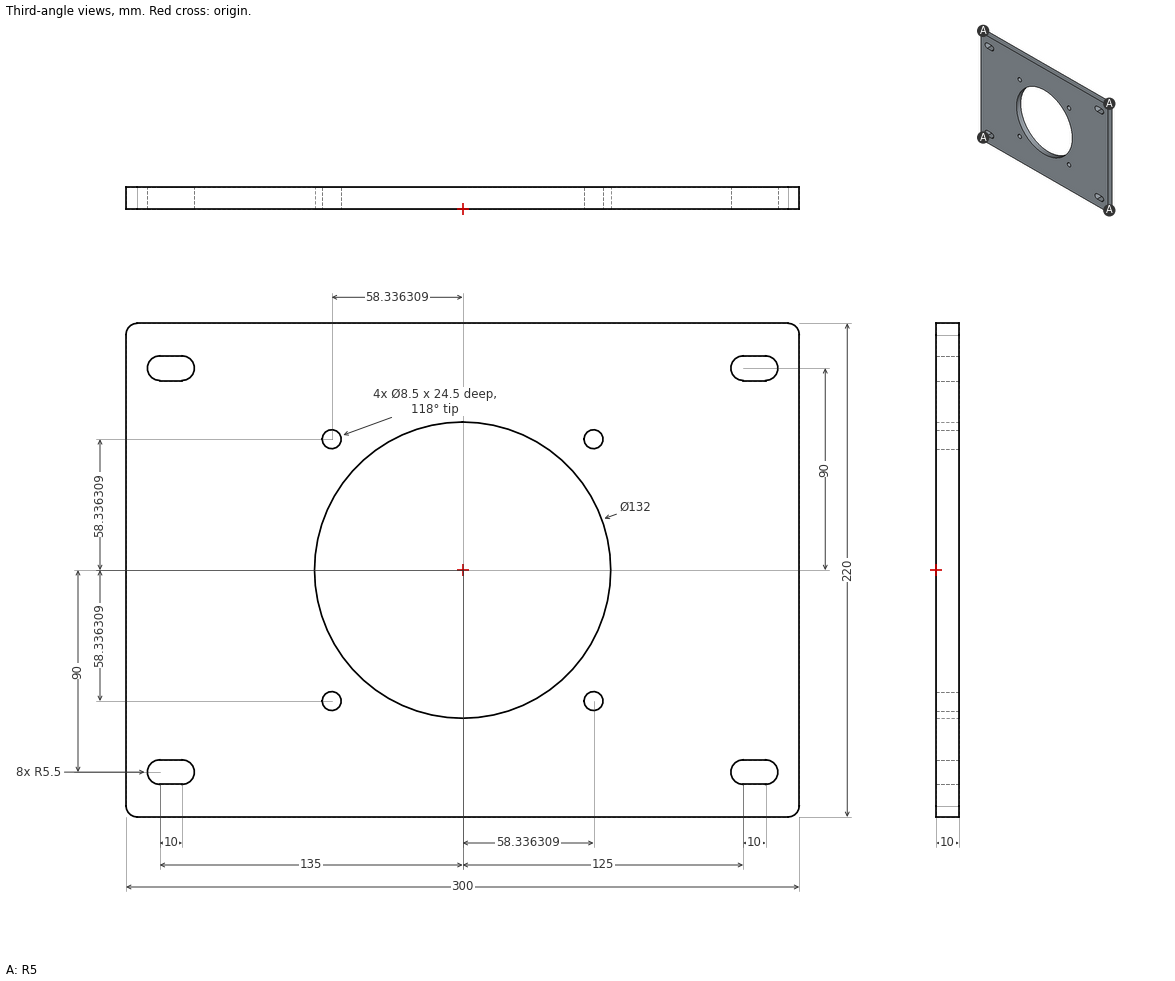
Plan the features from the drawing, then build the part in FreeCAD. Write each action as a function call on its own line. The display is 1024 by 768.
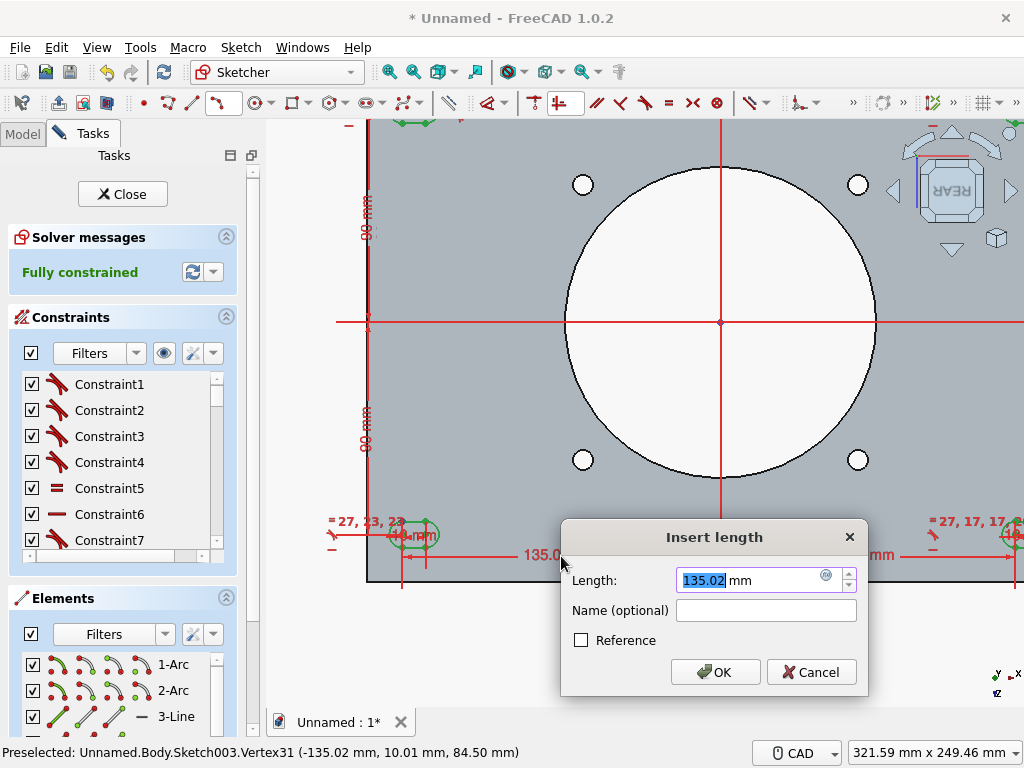
text(135)
key(Return)
key(Escape)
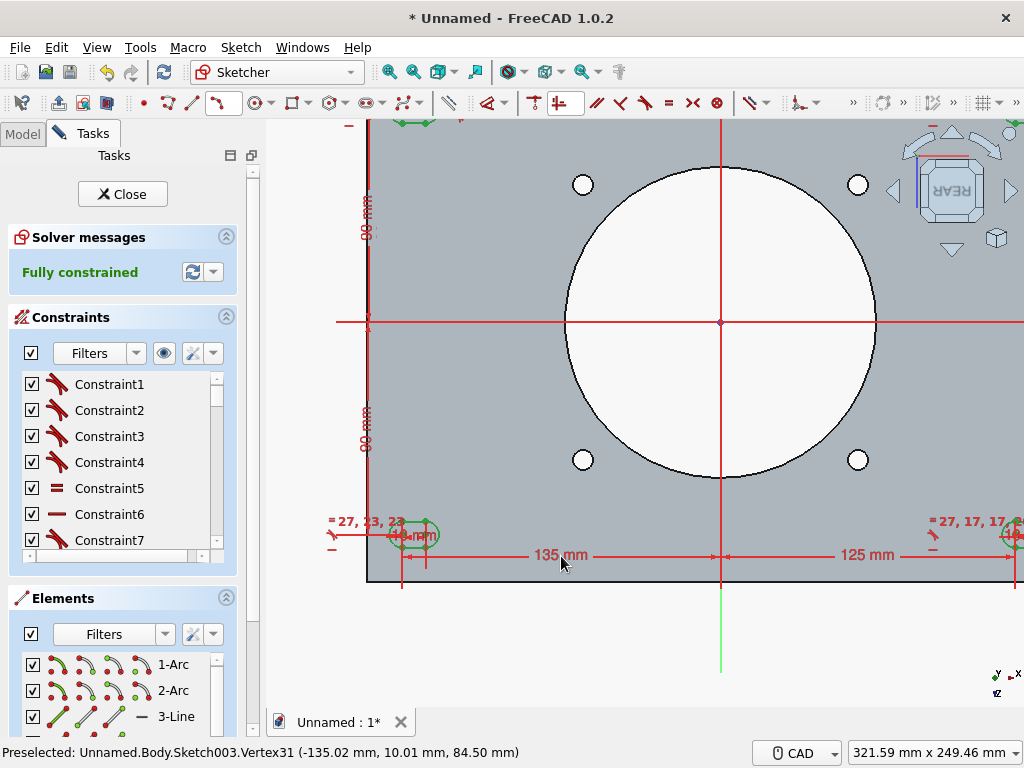
click(123, 194)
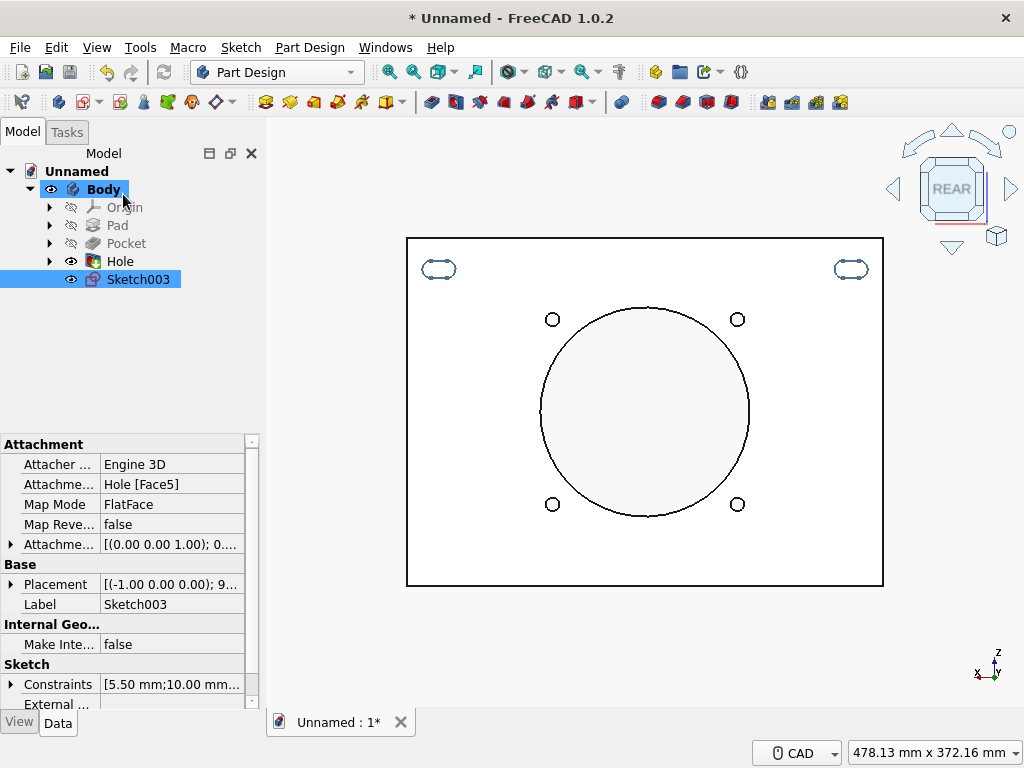
click(432, 102)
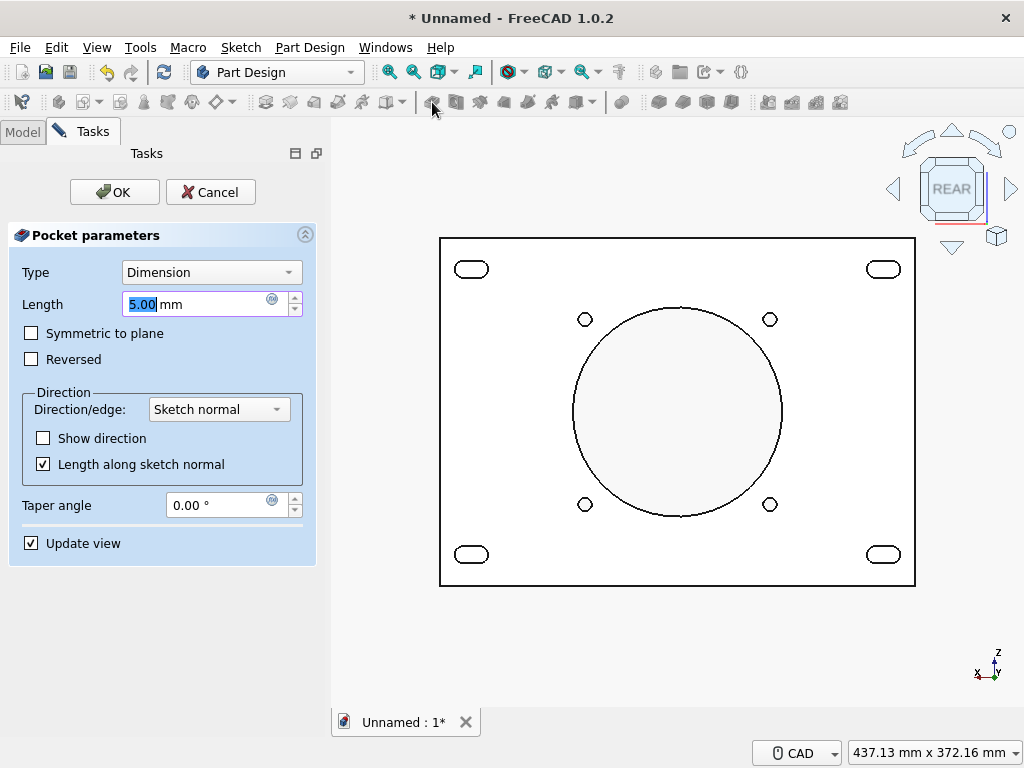
click(212, 272)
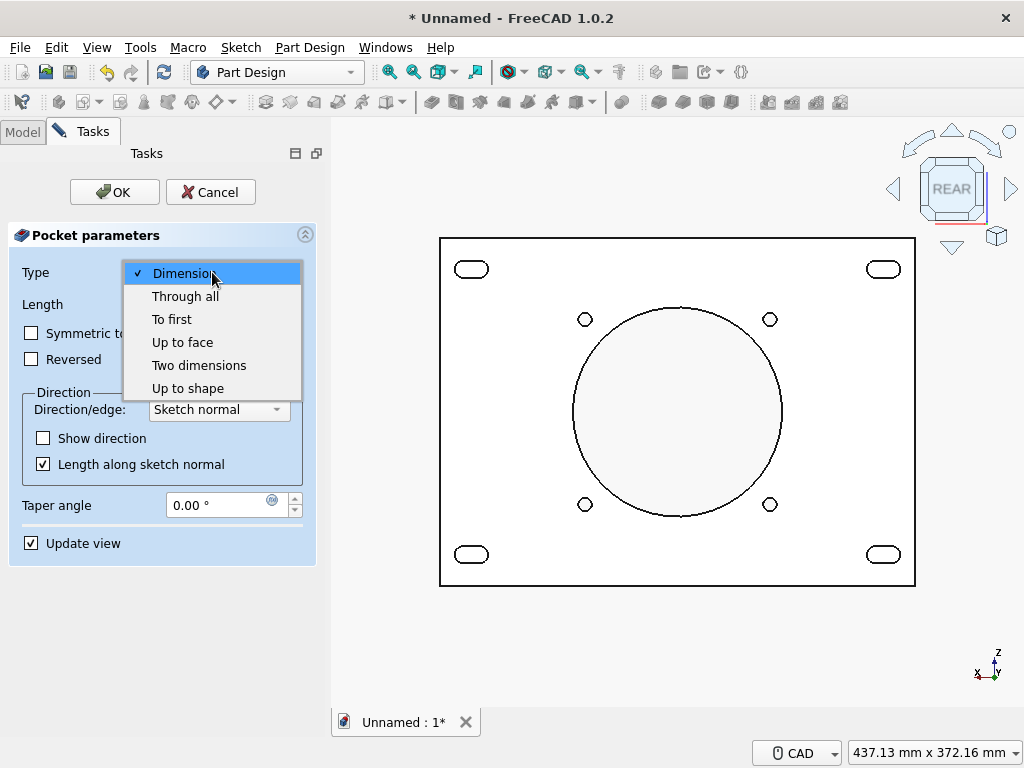
click(212, 296)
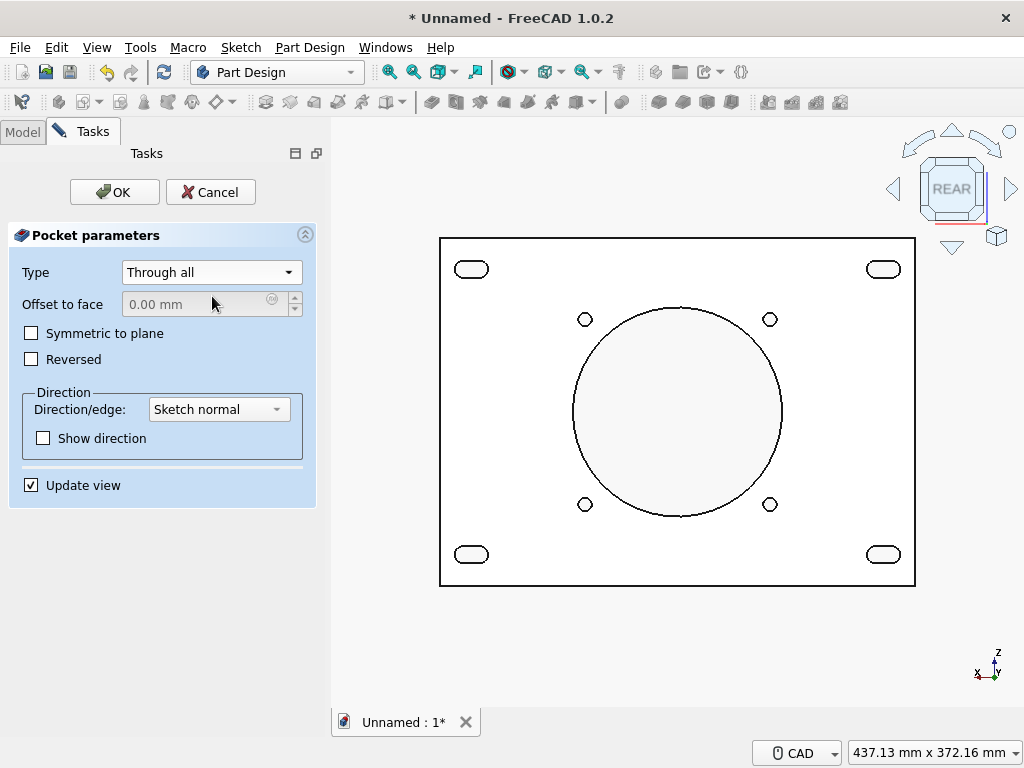
click(115, 192)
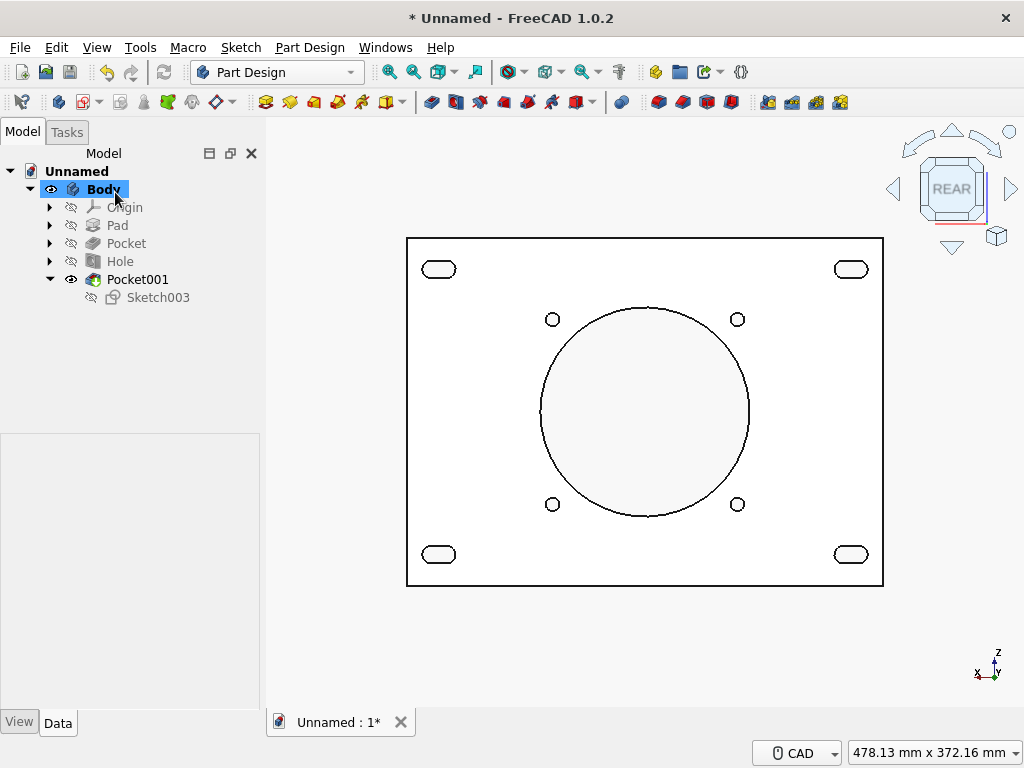
scroll(407, 237, up, 5)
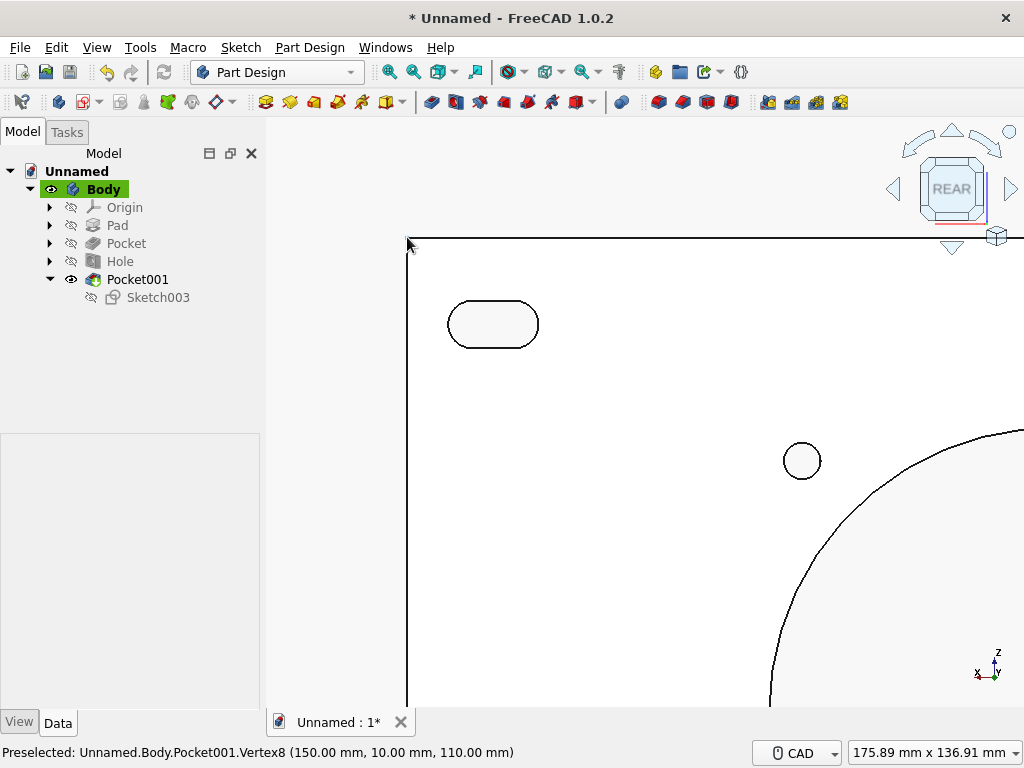
click(390, 72)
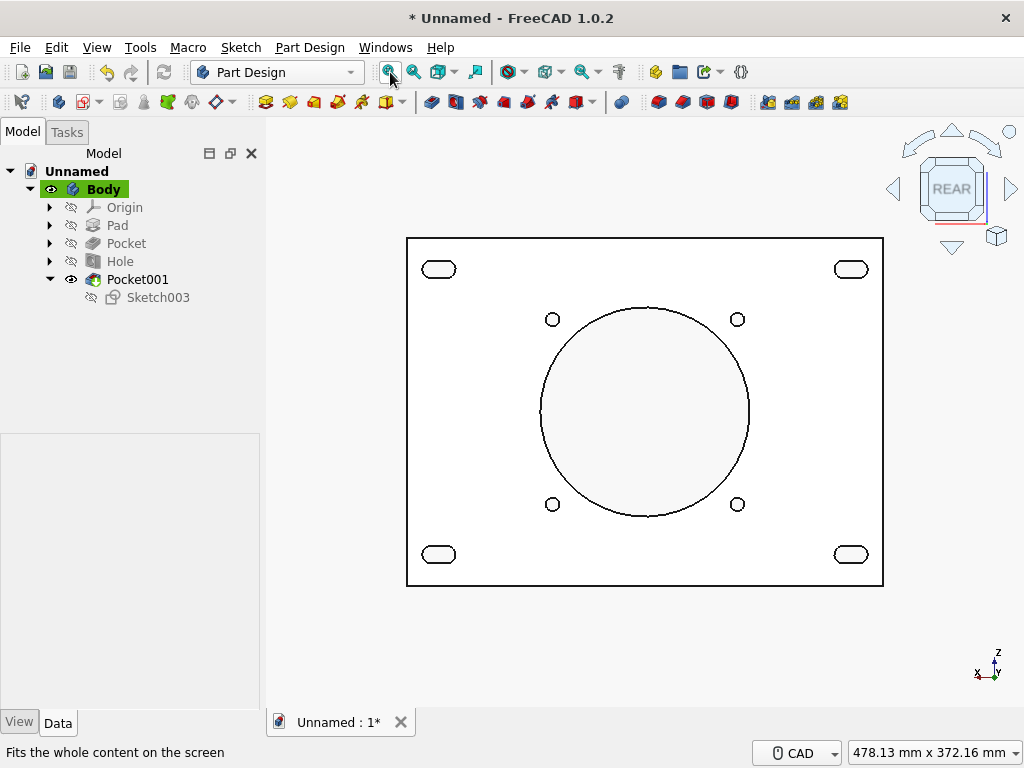
key(0)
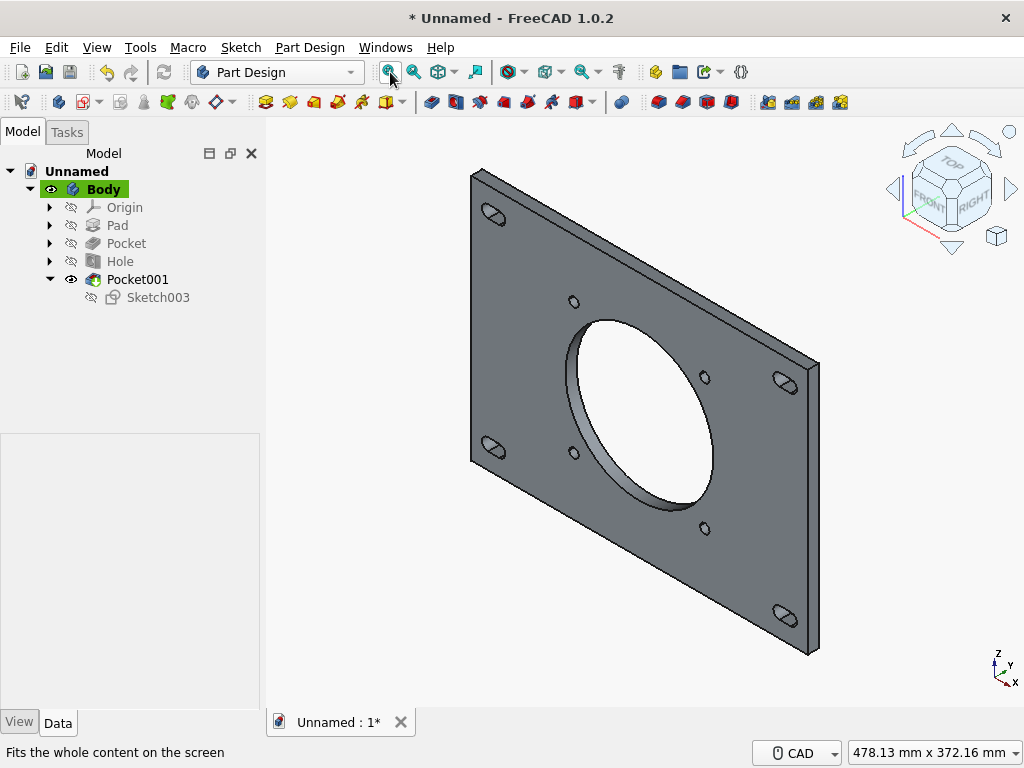
click(814, 365)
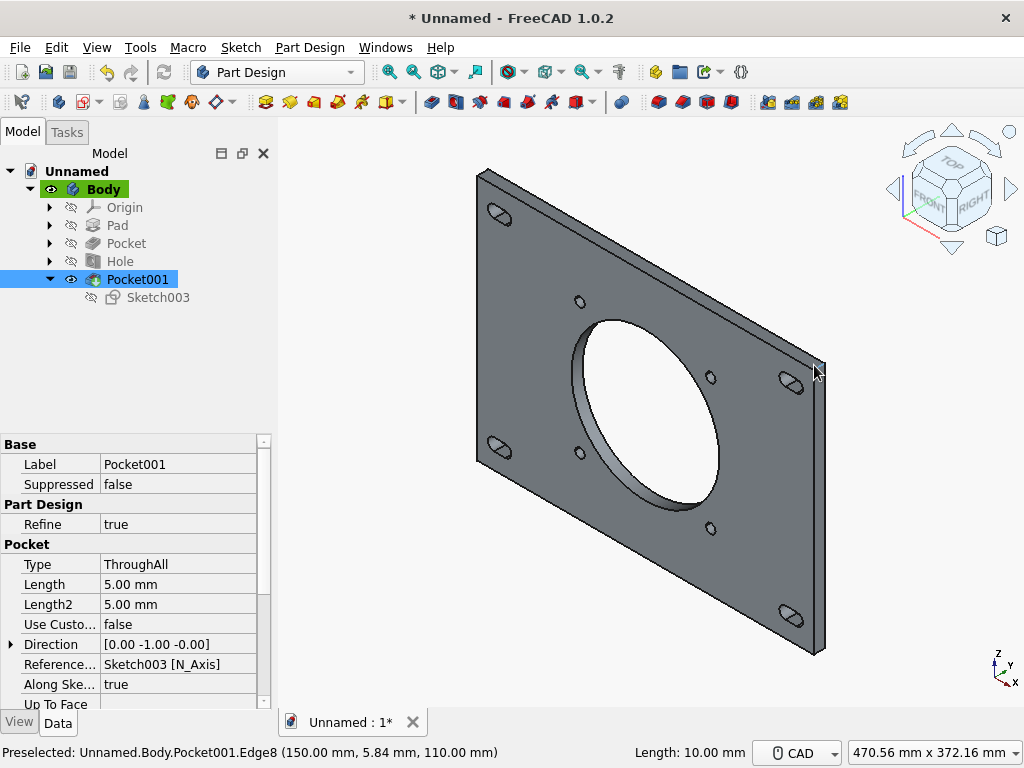
scroll(483, 172, up, 5)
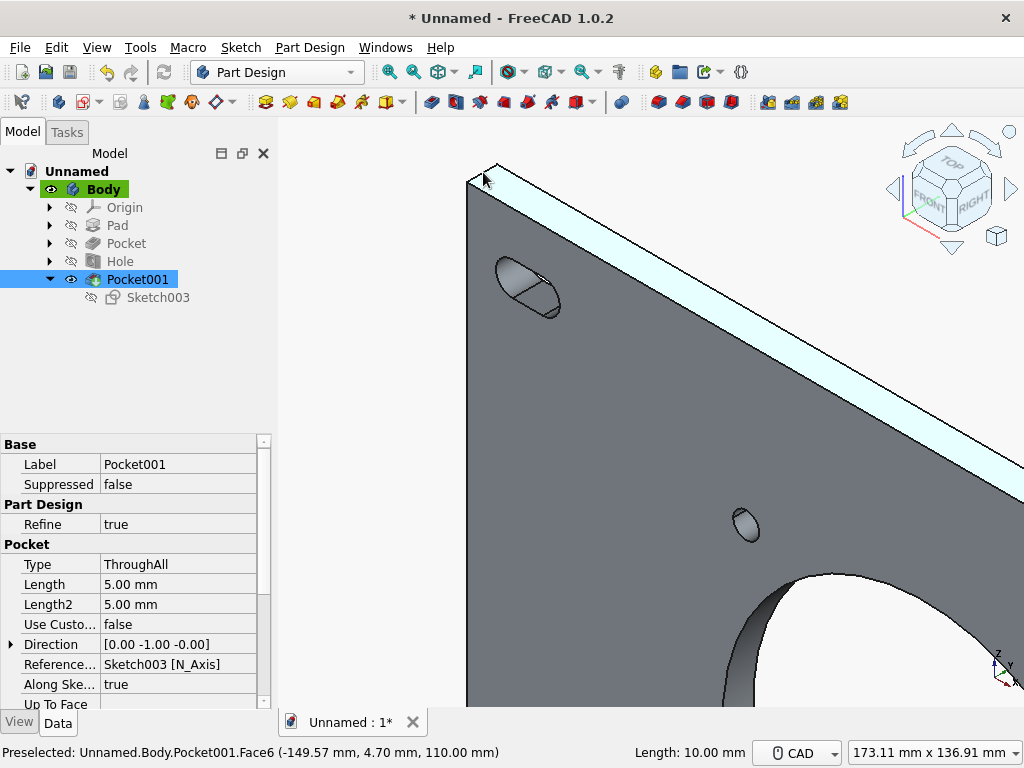
key(v)
key(f)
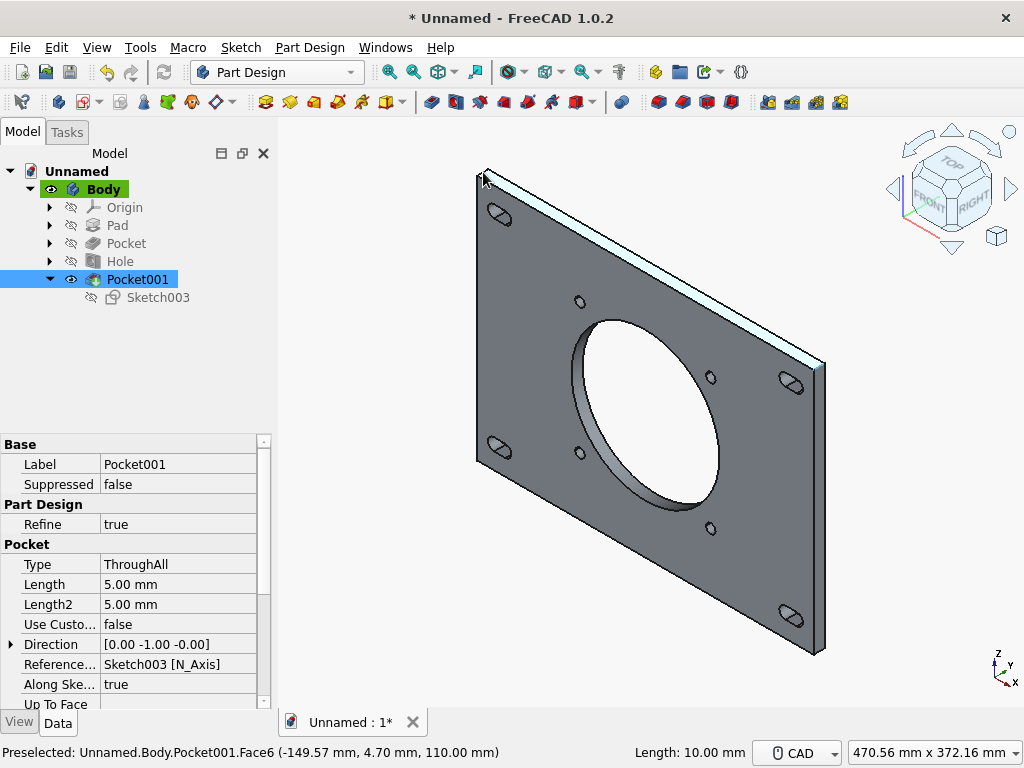
key(2)